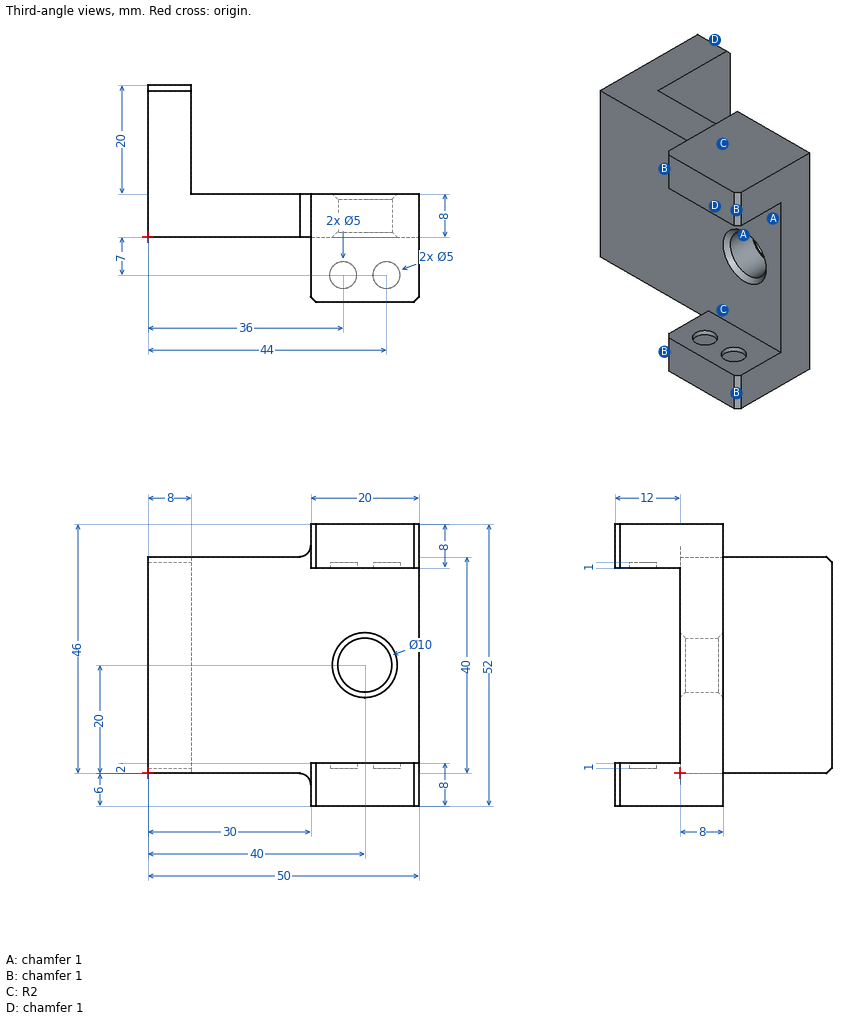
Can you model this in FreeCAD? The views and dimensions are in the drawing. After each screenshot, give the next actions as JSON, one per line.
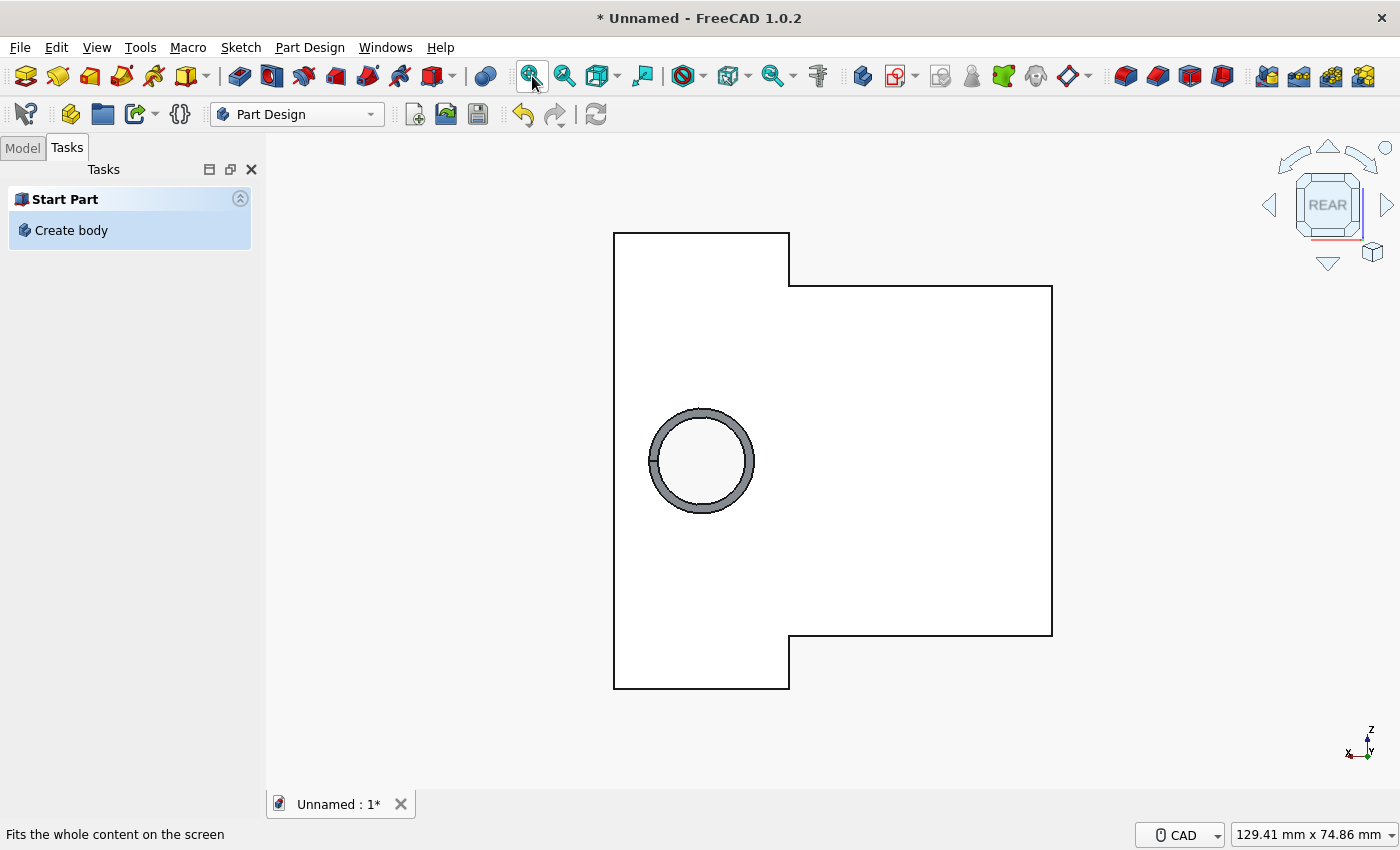
{"action": "key", "text": "6"}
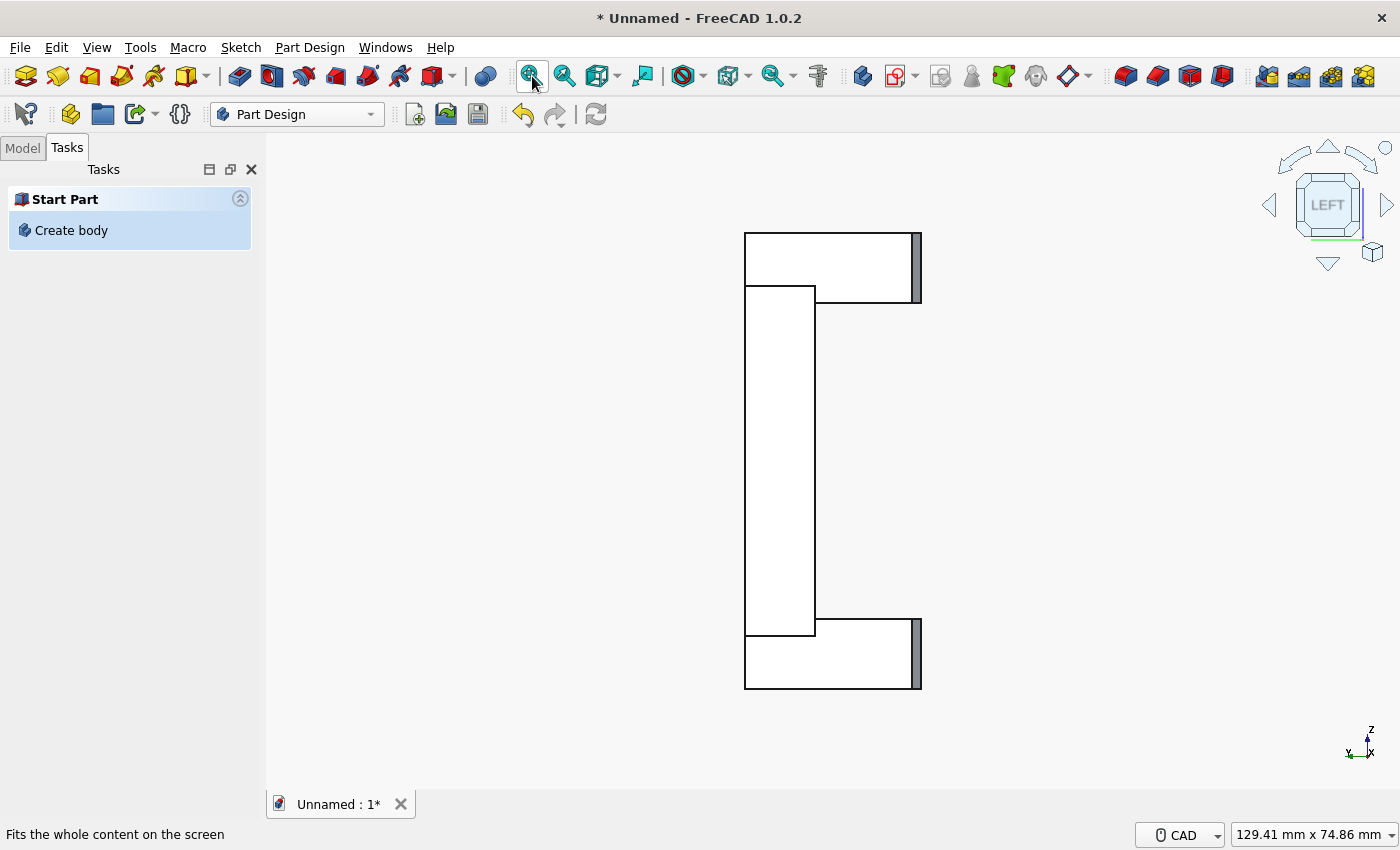
{"action": "key", "text": "v 3"}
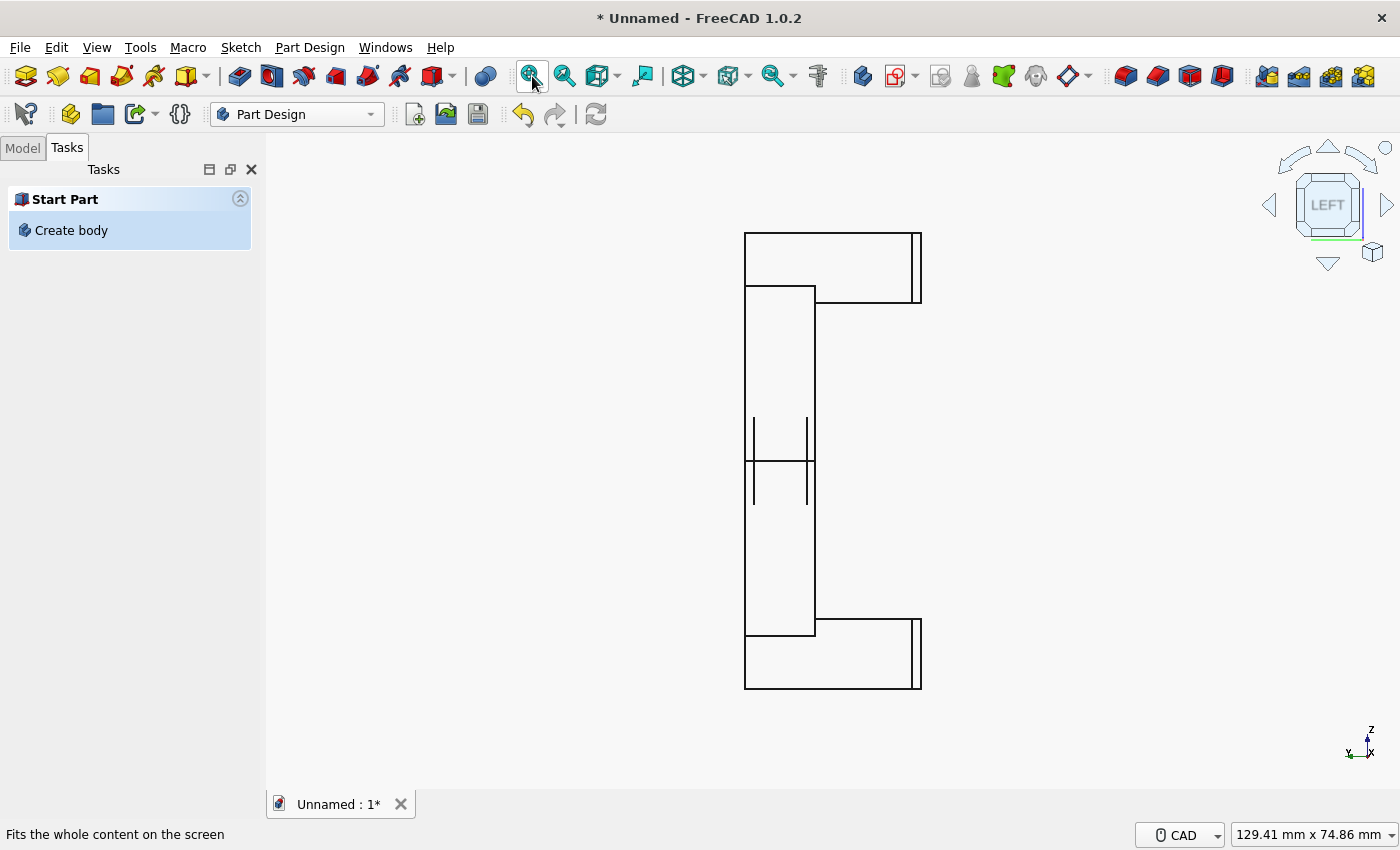
{"action": "key", "text": "0"}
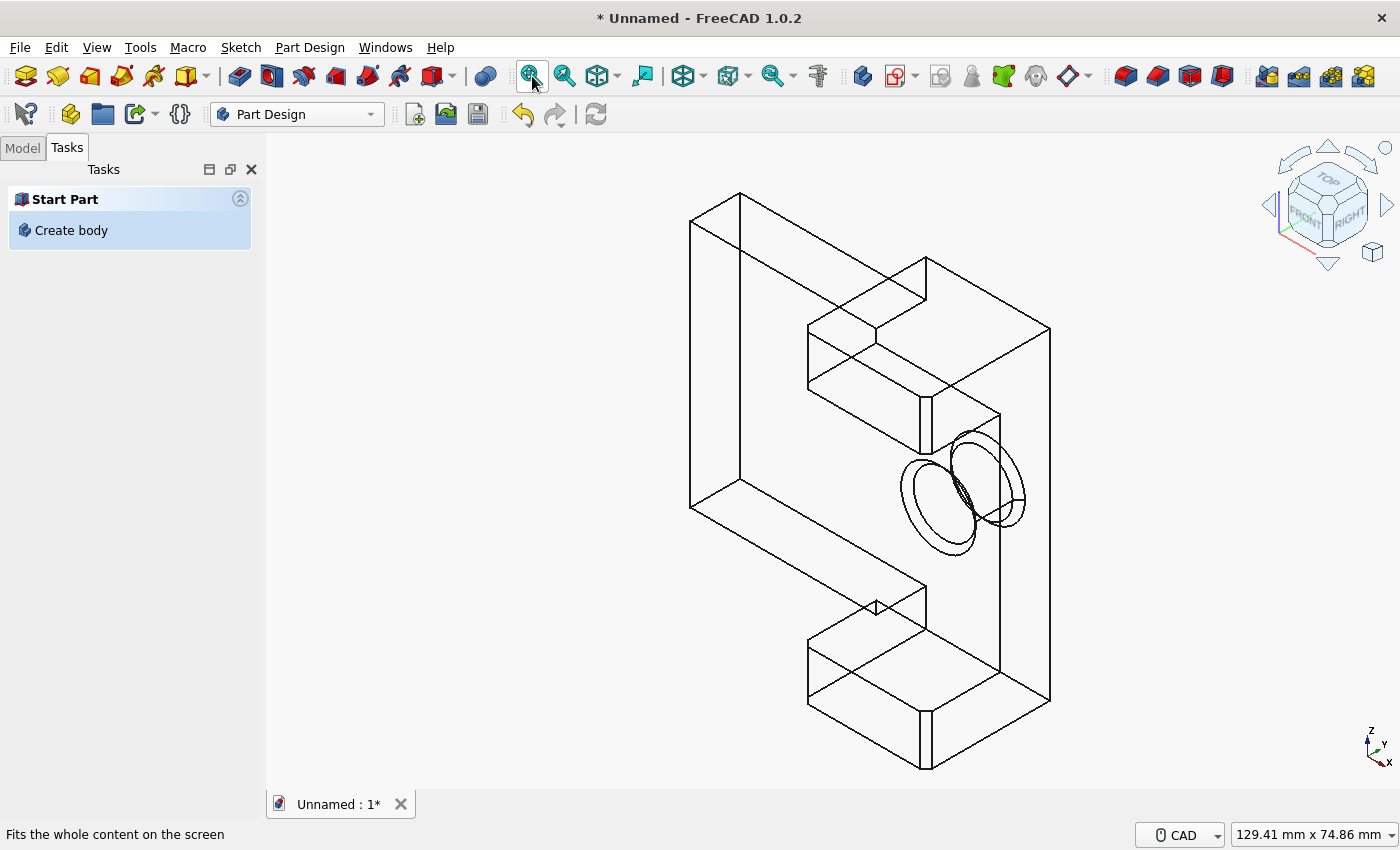
{"action": "left_click", "coordinate": [901, 313]}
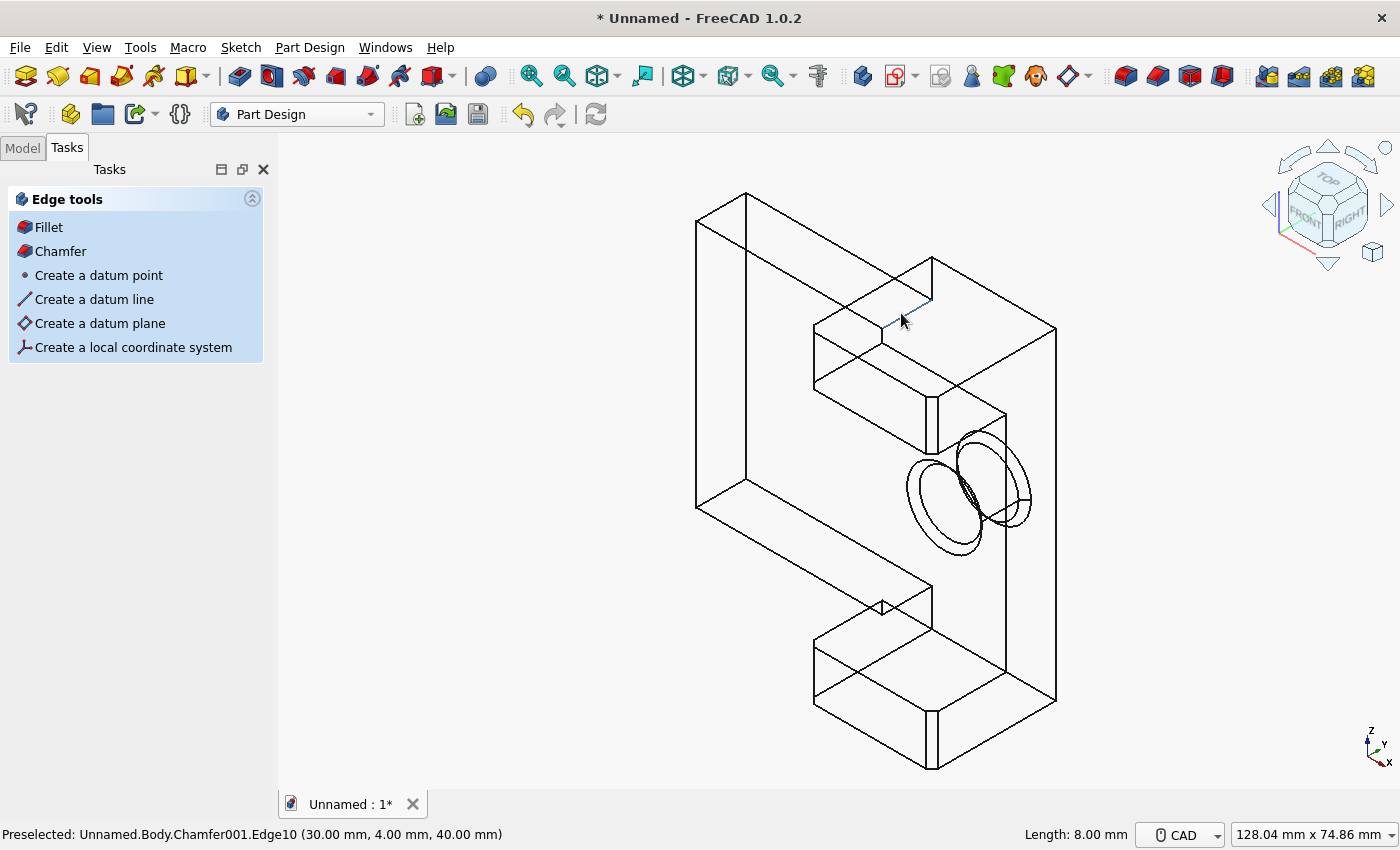
{"action": "left_click", "coordinate": [907, 600], "text": "ctrl"}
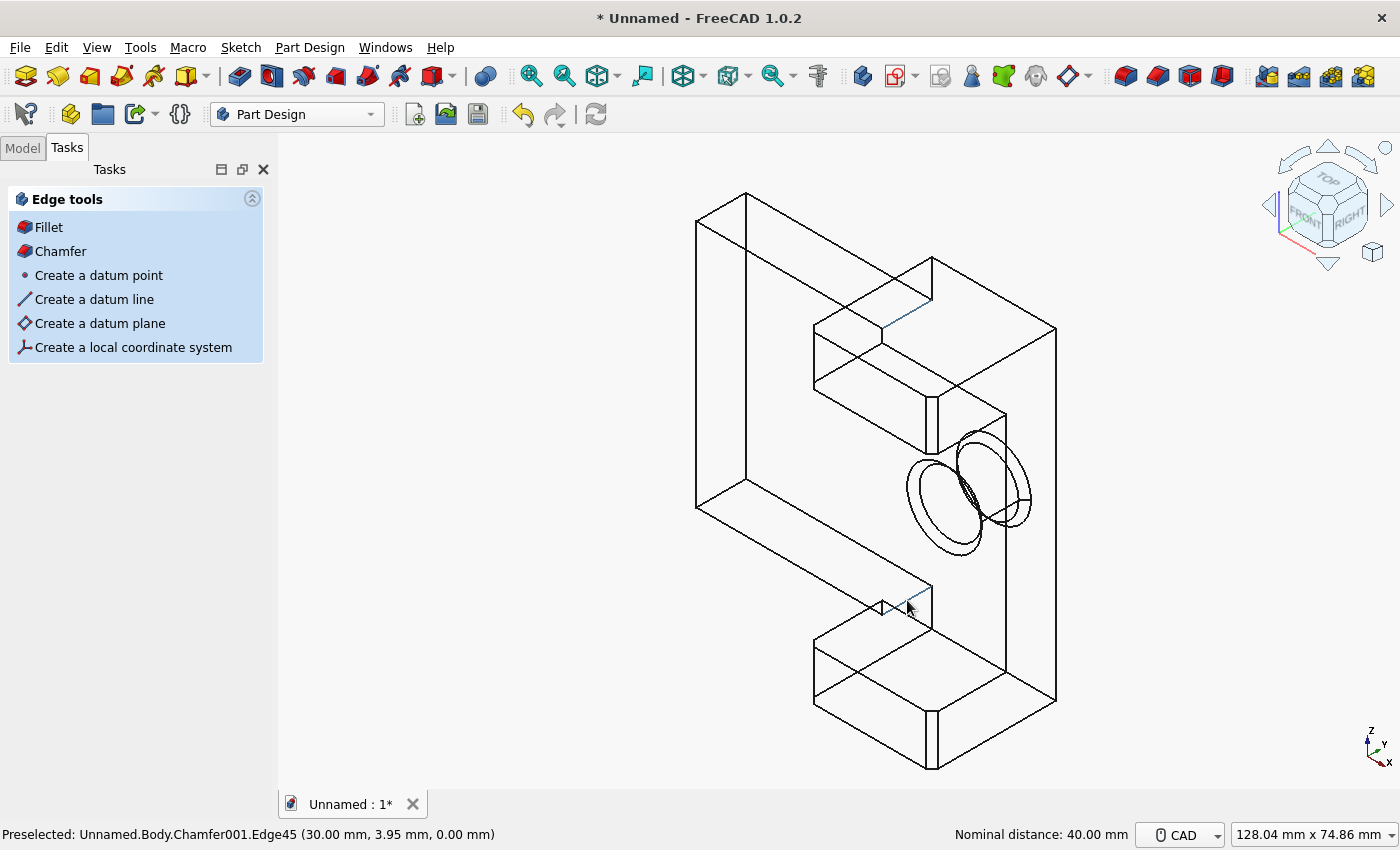
{"action": "key", "text": "v 1"}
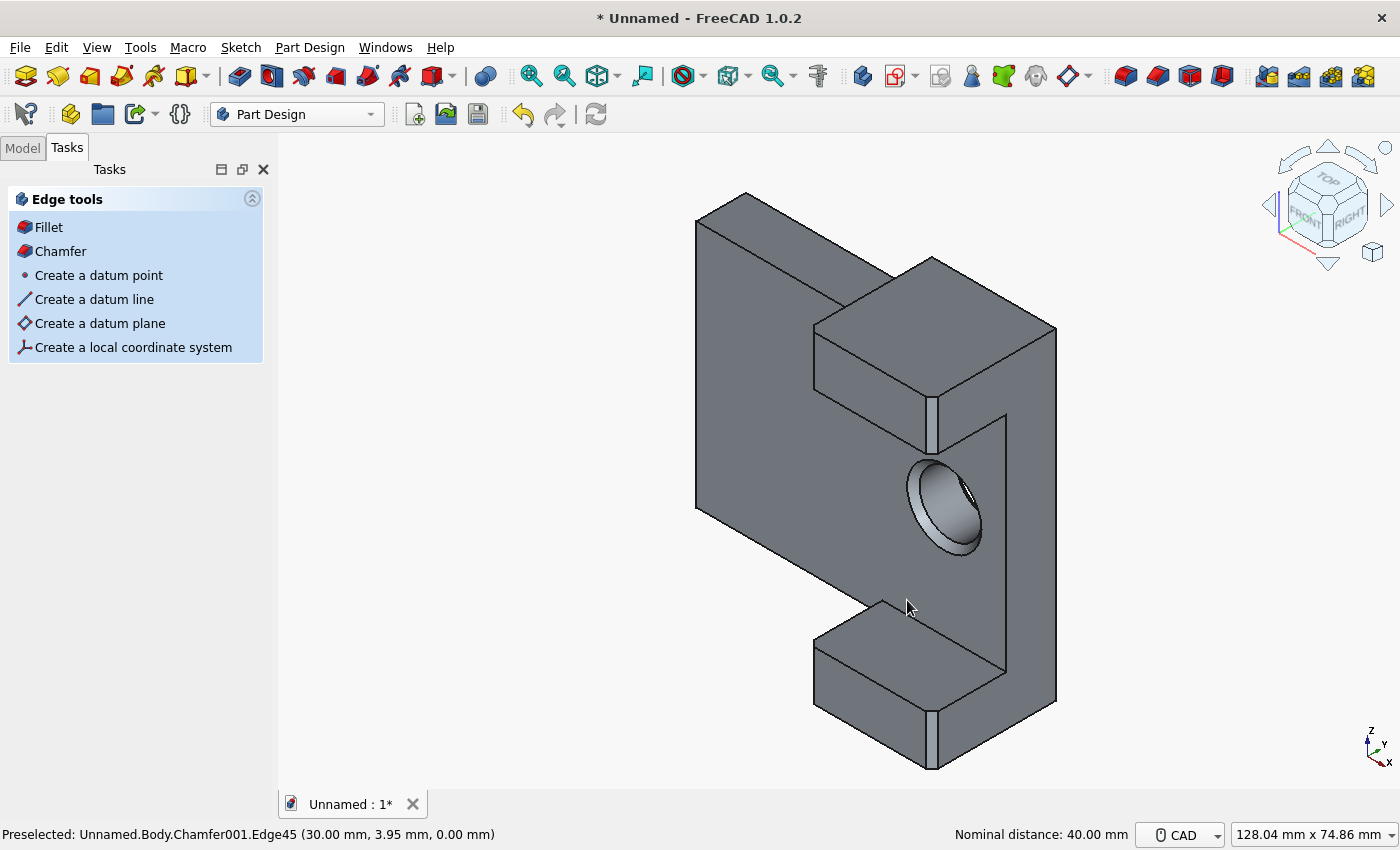
{"action": "left_click", "coordinate": [1126, 76]}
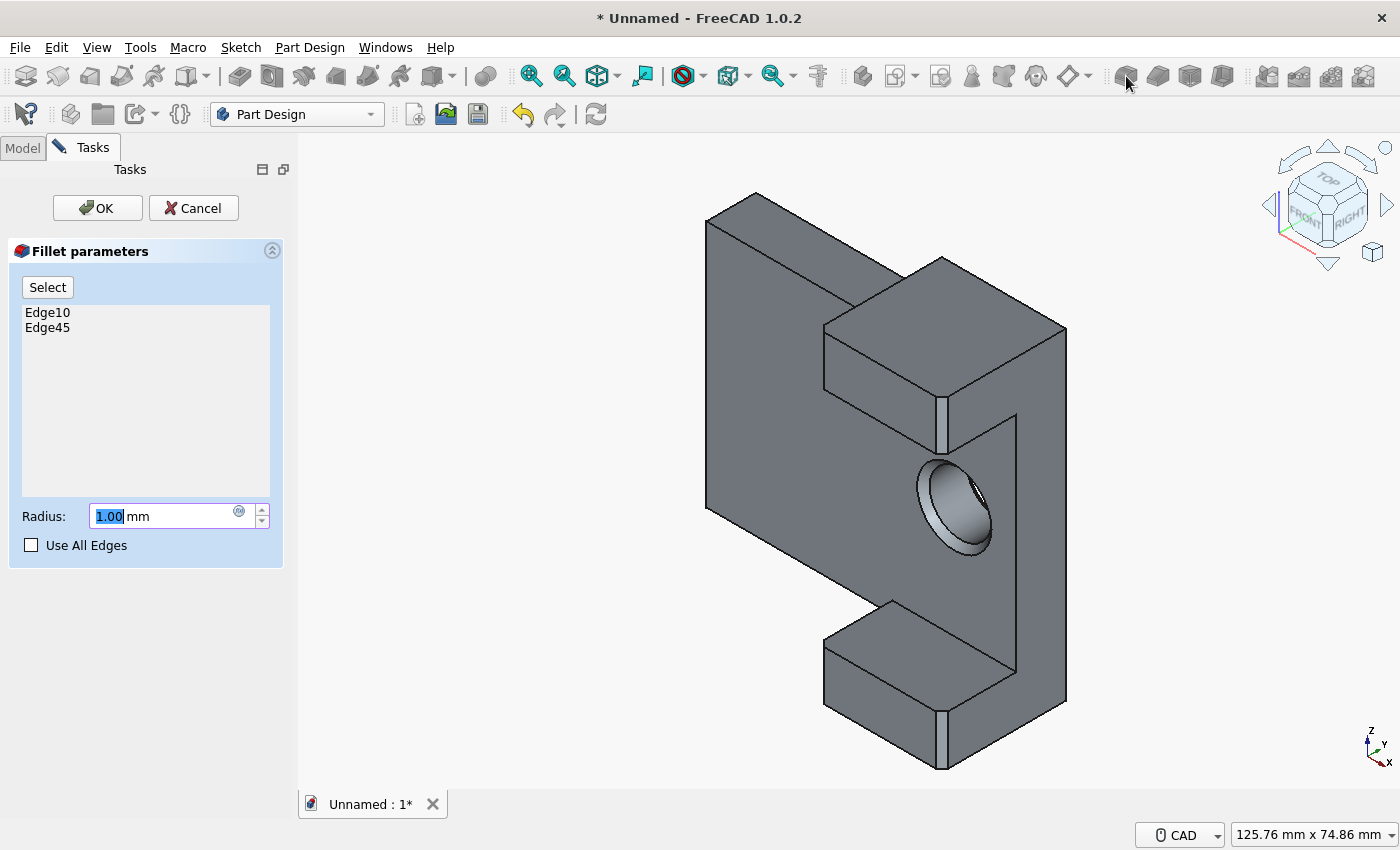
{"action": "type", "text": "2"}
{"action": "key", "text": "Tab"}